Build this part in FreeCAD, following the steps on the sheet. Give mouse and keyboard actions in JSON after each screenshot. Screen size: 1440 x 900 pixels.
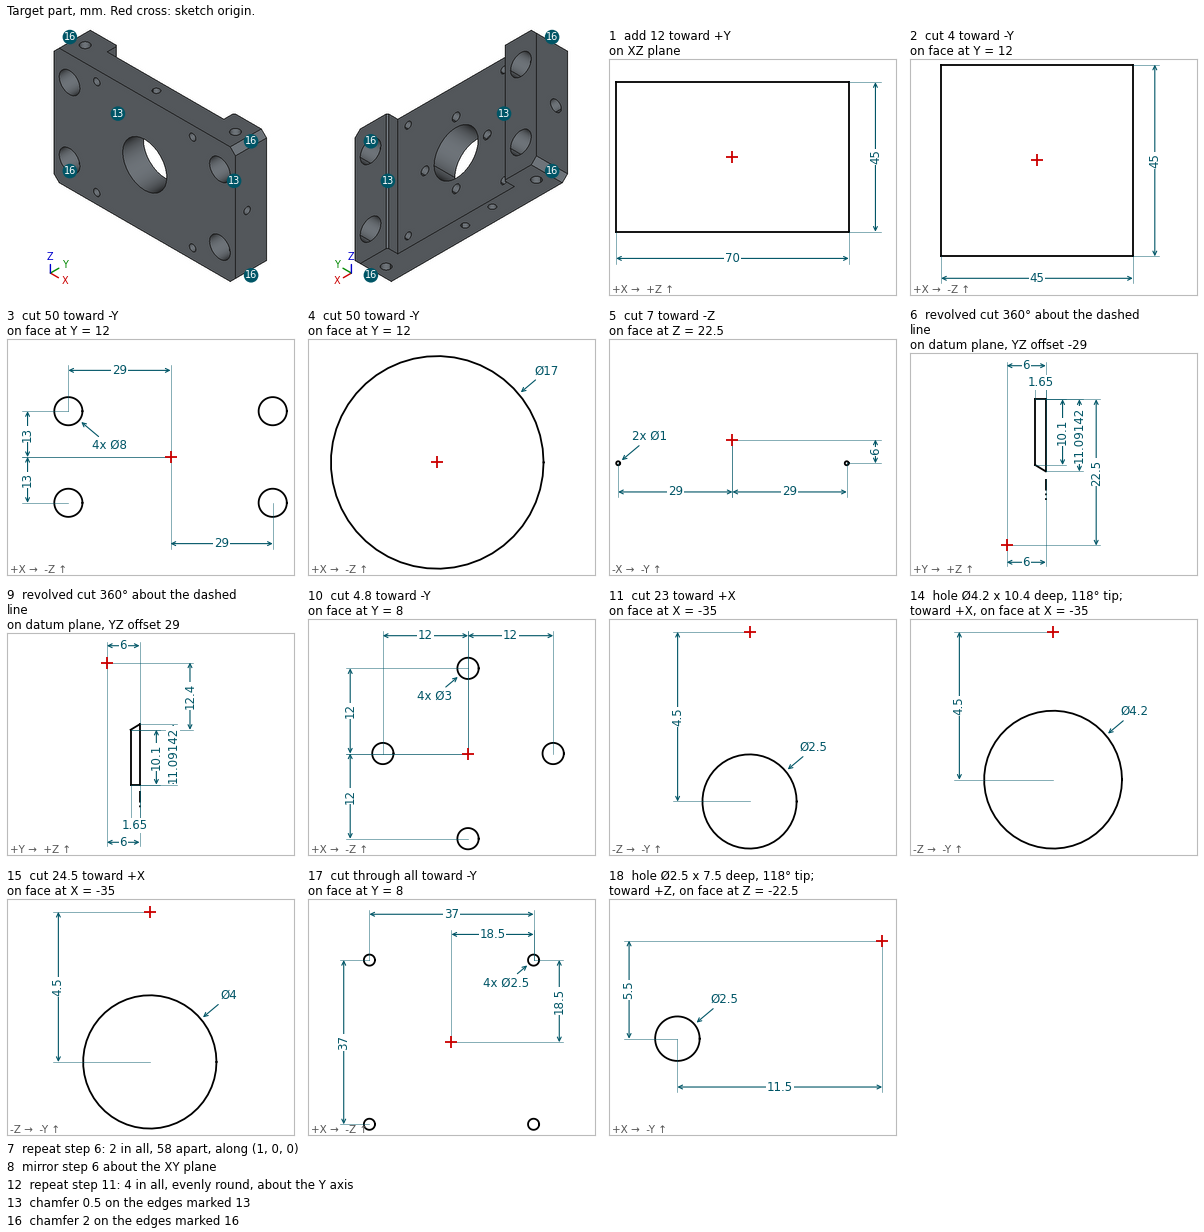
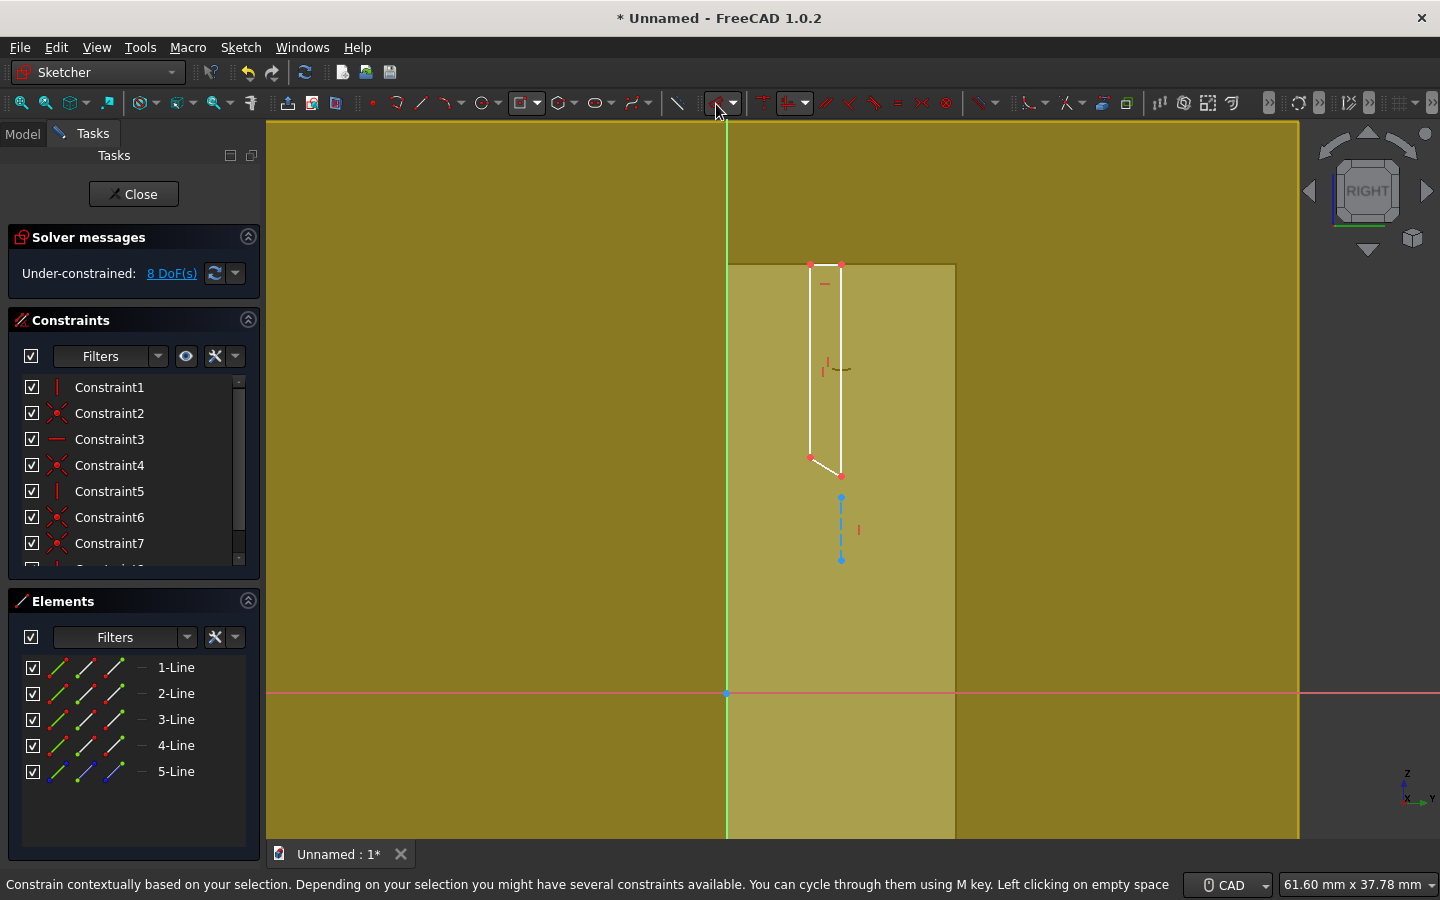
{"action": "left_click", "coordinate": [841, 477]}
{"action": "left_click", "coordinate": [784, 727]}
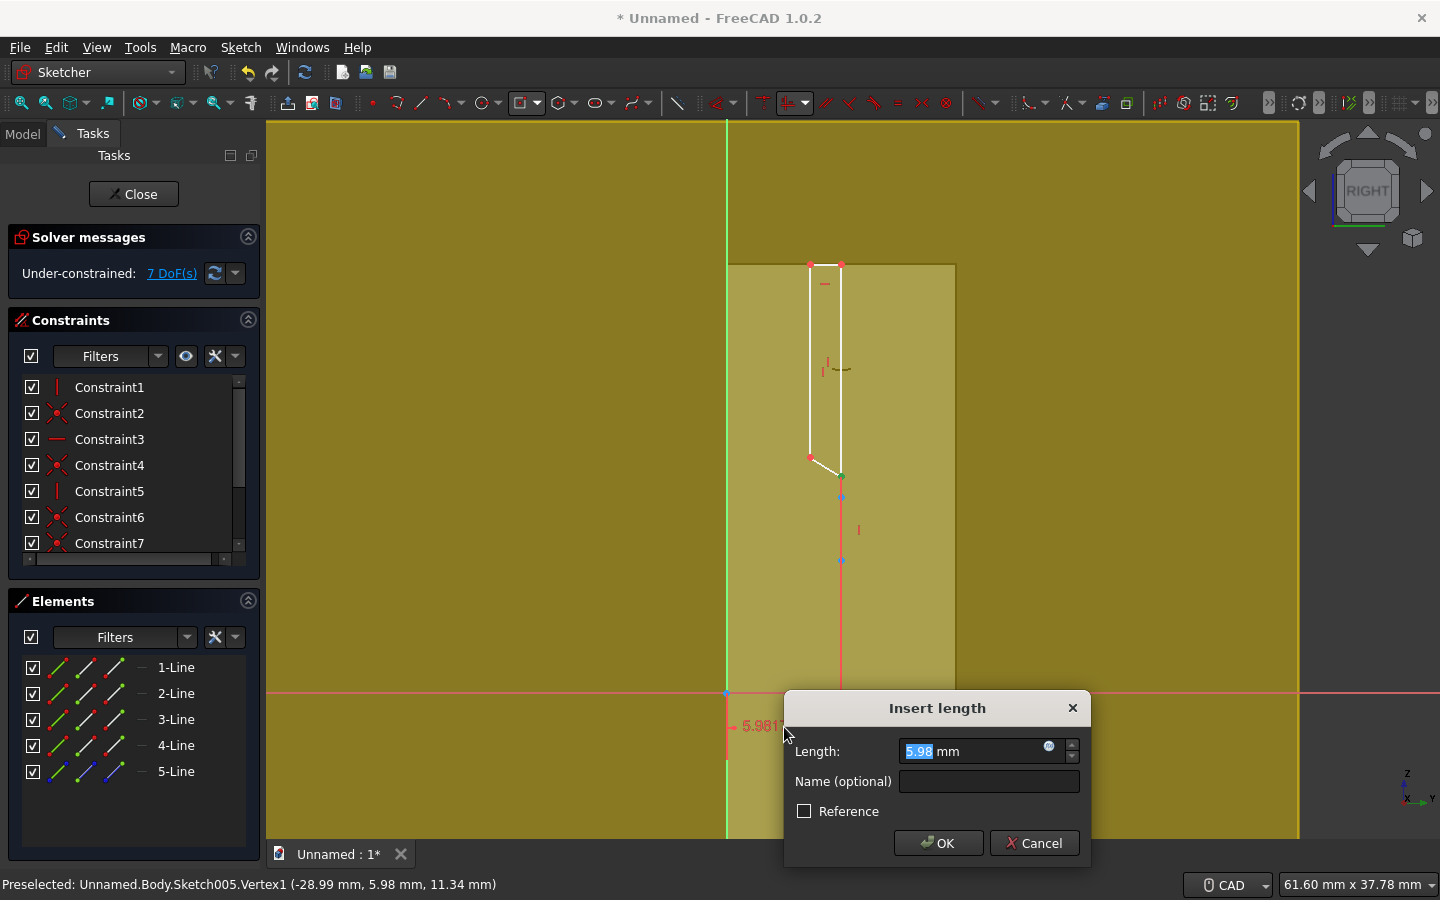
{"action": "type", "text": "6"}
{"action": "key", "text": "Return"}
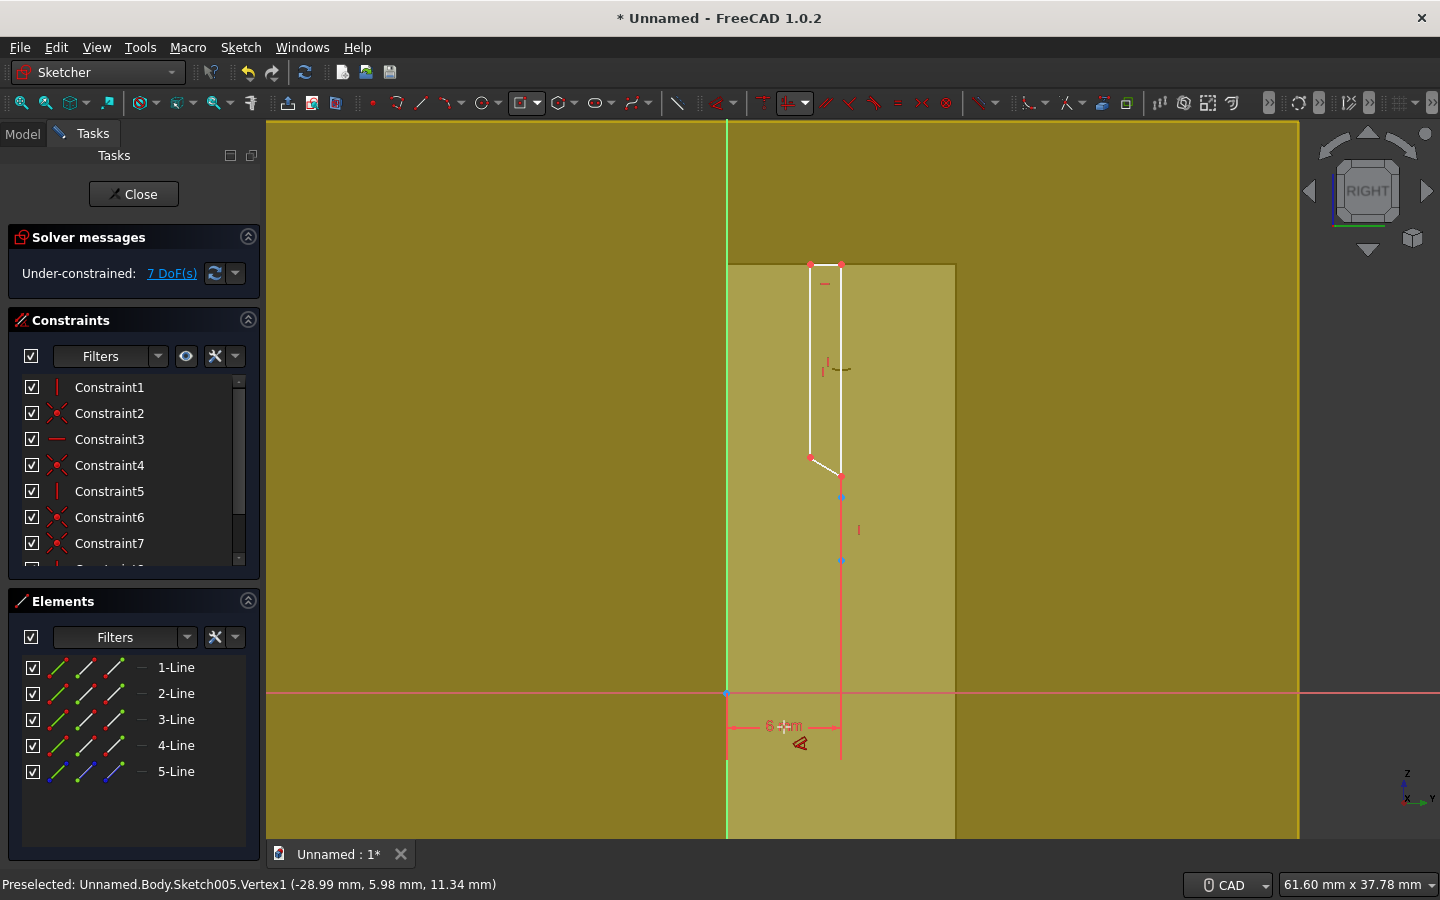
{"action": "left_click", "coordinate": [841, 498]}
{"action": "left_click", "coordinate": [784, 464]}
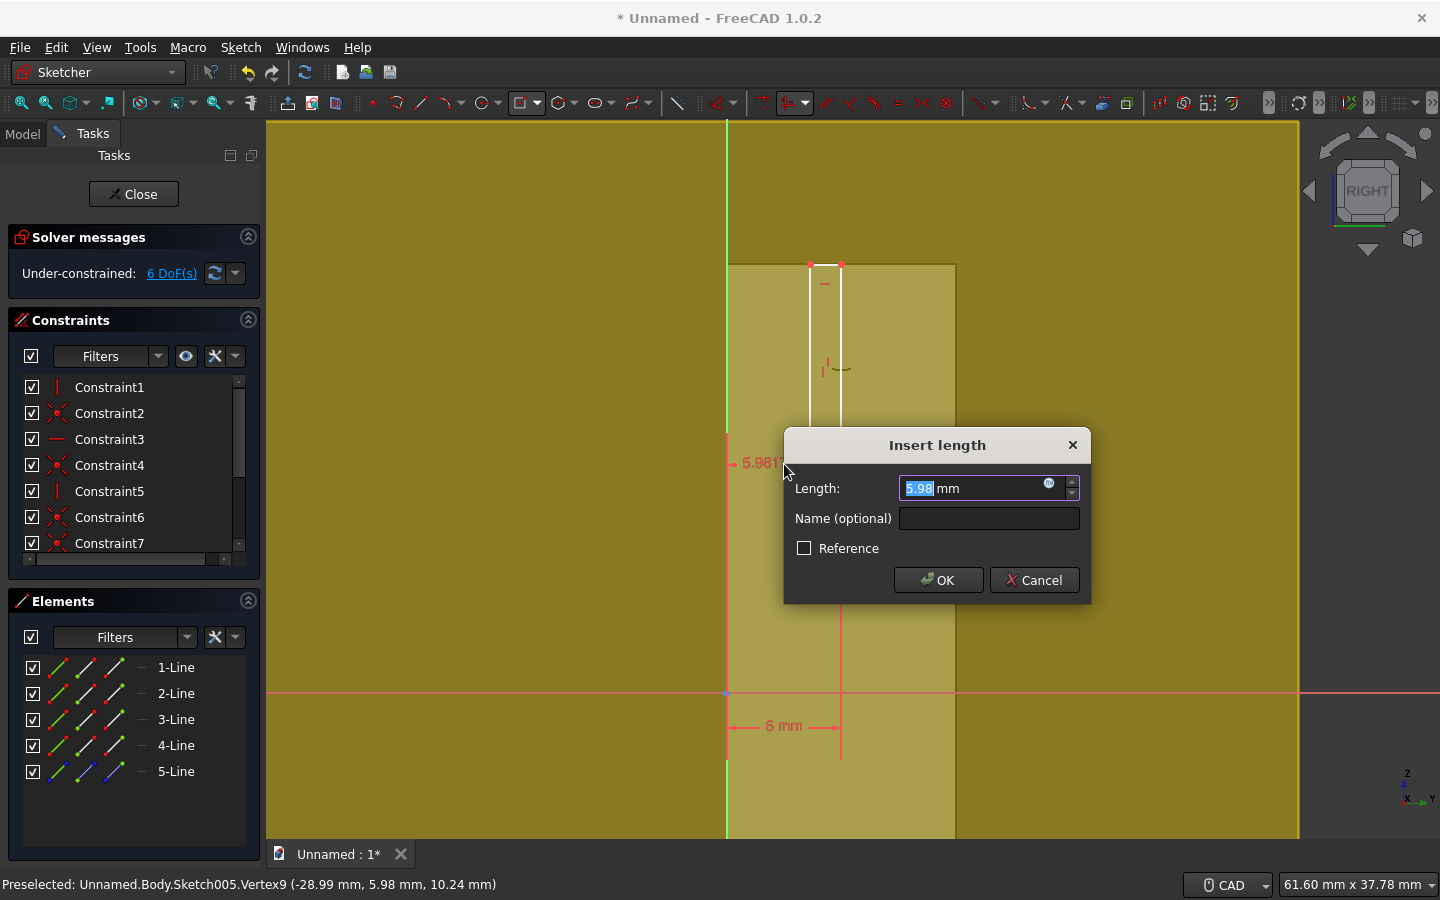
{"action": "type", "text": "6"}
{"action": "key", "text": "Return"}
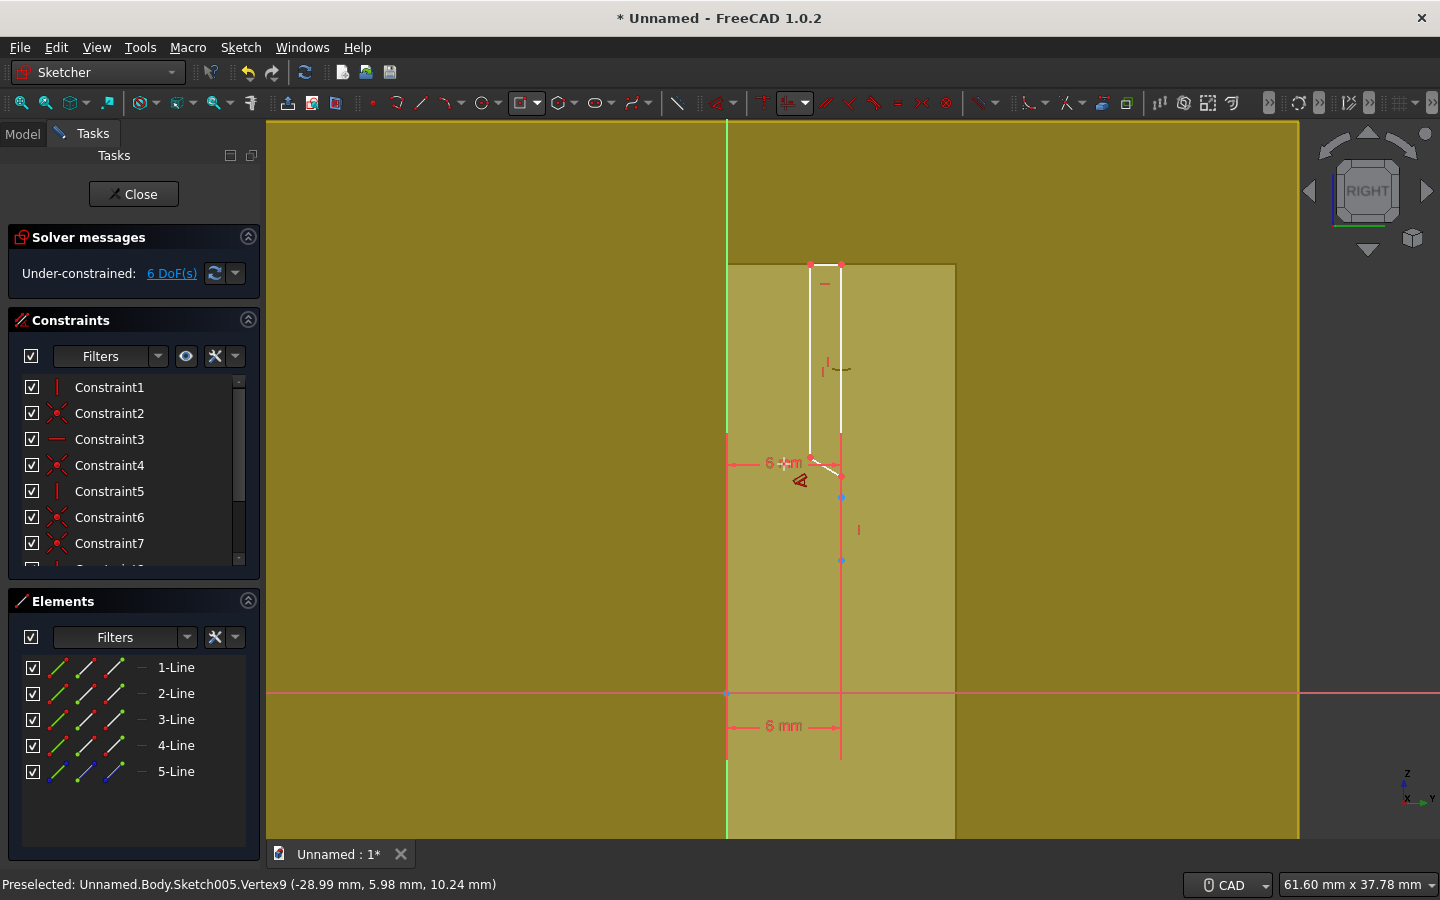
{"action": "scroll", "coordinate": [832, 265], "scroll_direction": "up", "scroll_amount": 2}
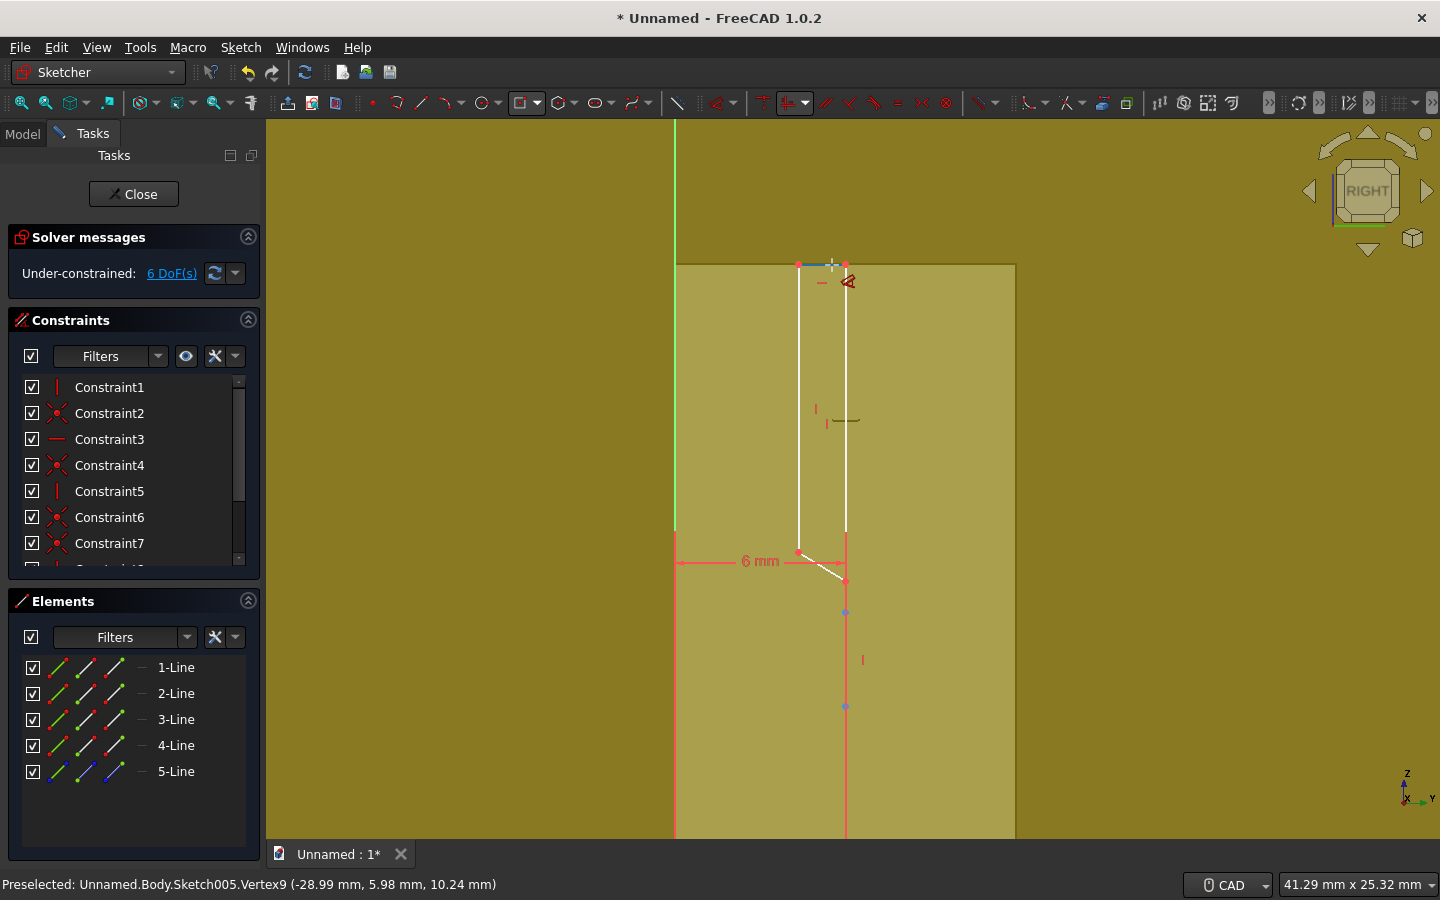
{"action": "left_click", "coordinate": [832, 265]}
{"action": "left_click", "coordinate": [822, 231]}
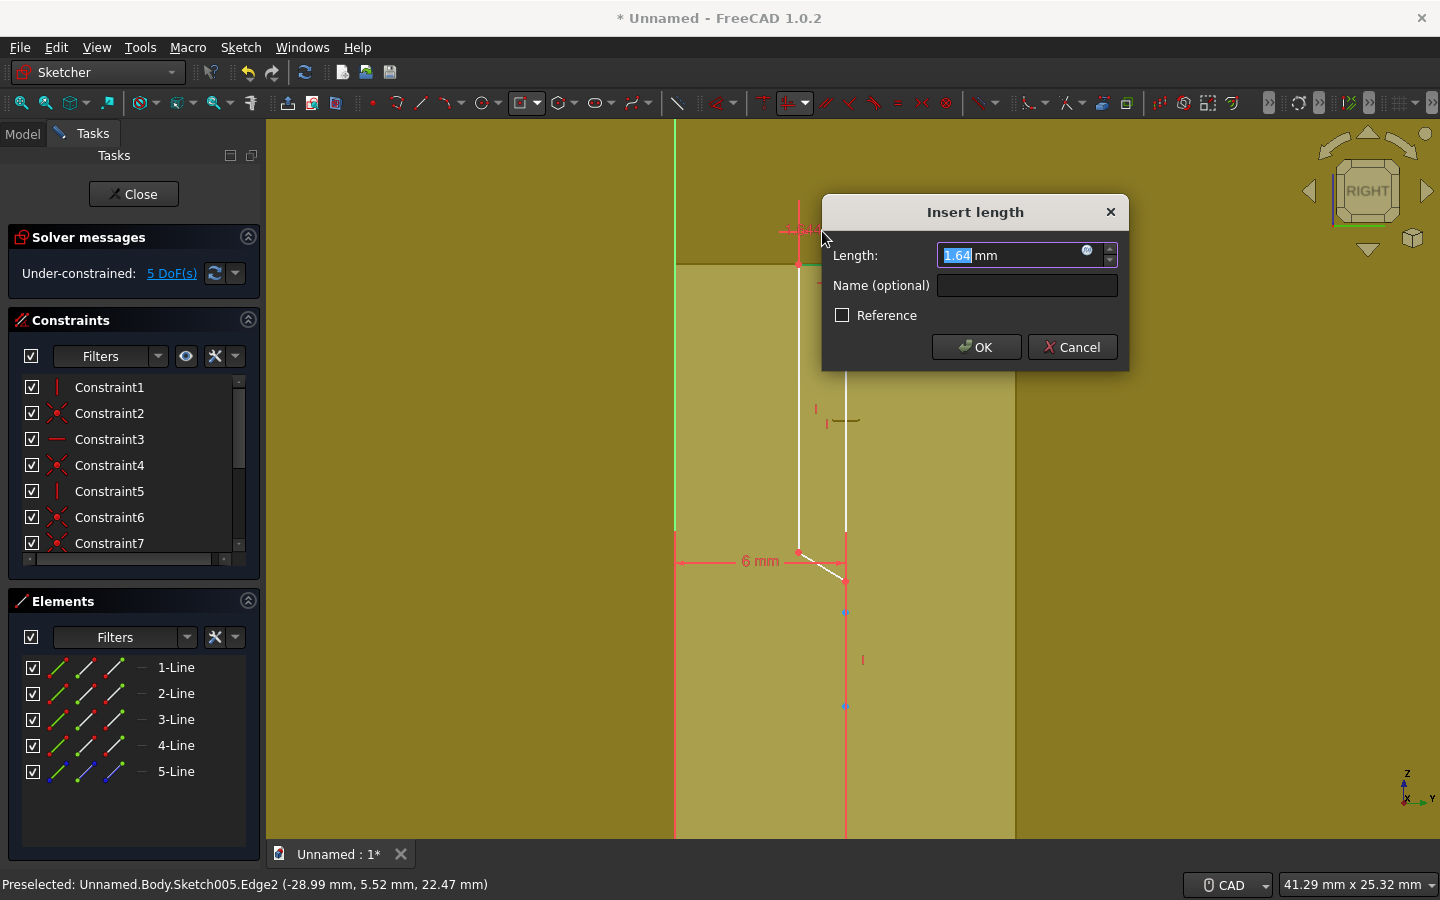
{"action": "type", "text": "1.65"}
{"action": "key", "text": "Return"}